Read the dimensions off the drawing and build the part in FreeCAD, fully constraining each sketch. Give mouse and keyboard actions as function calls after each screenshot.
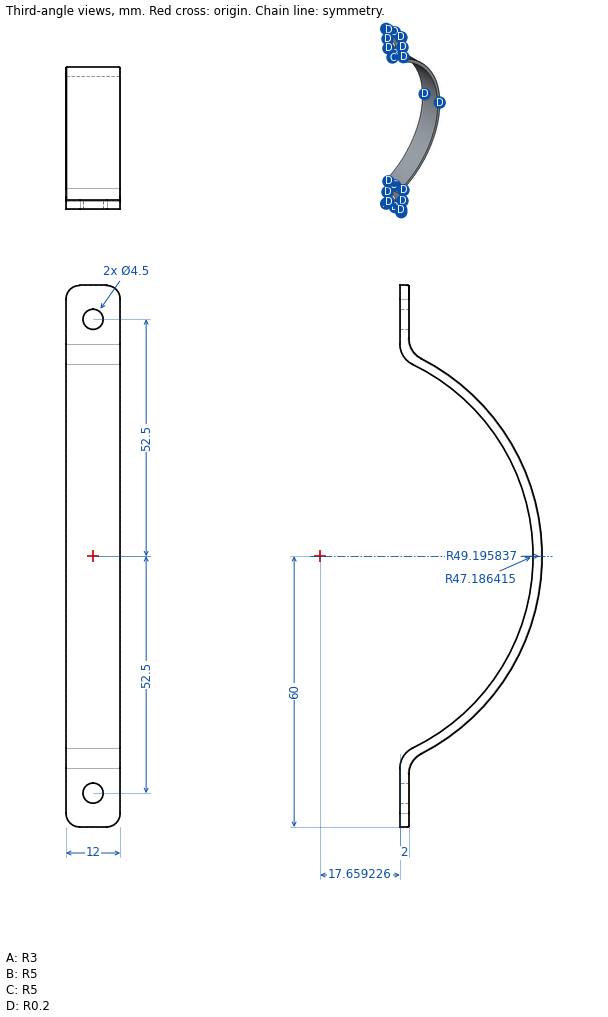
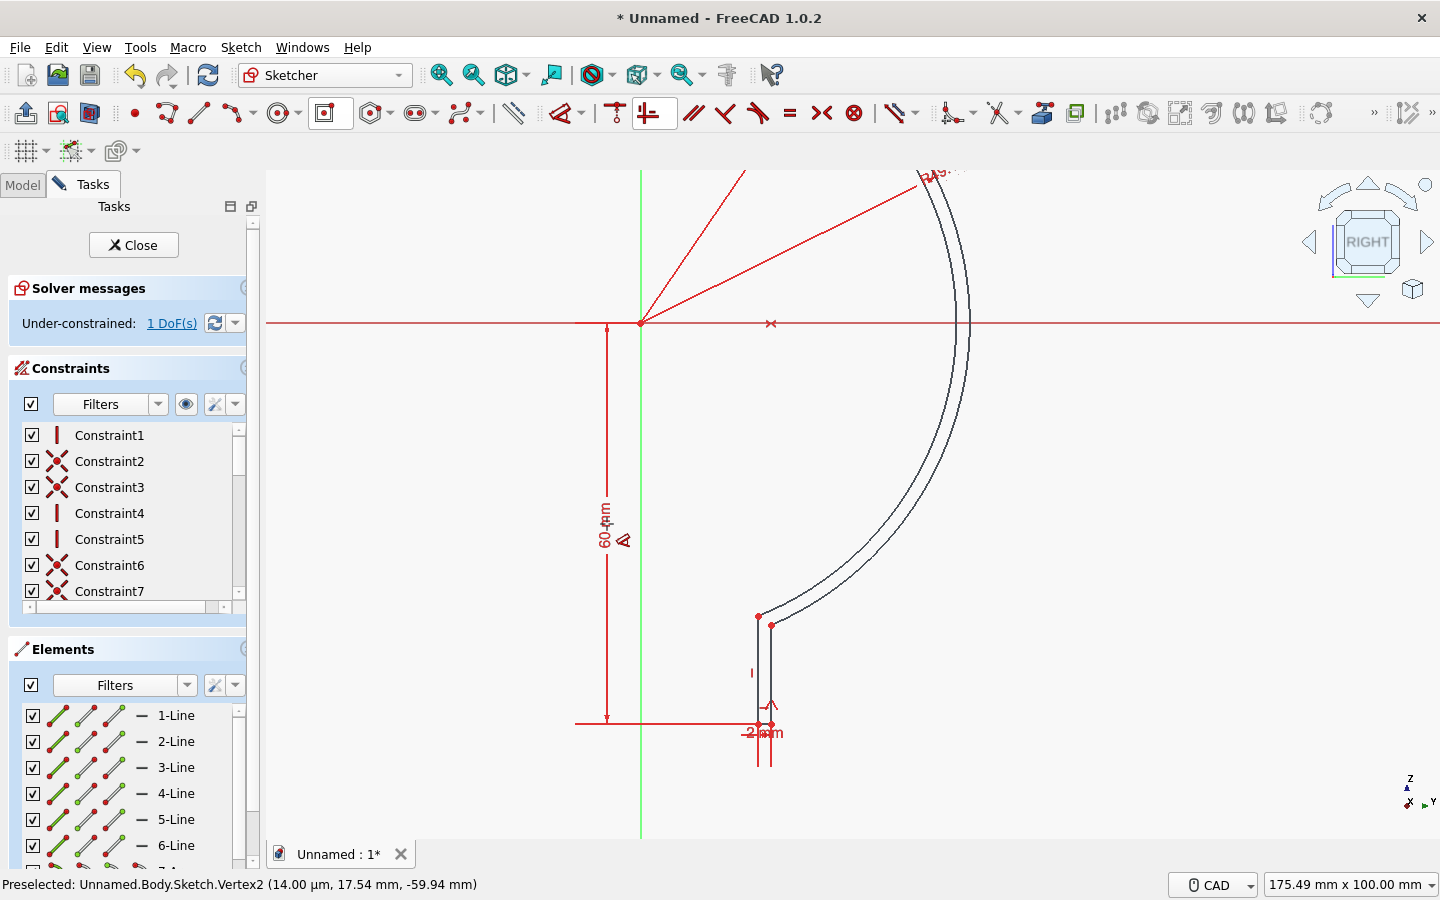
click(758, 616)
click(699, 650)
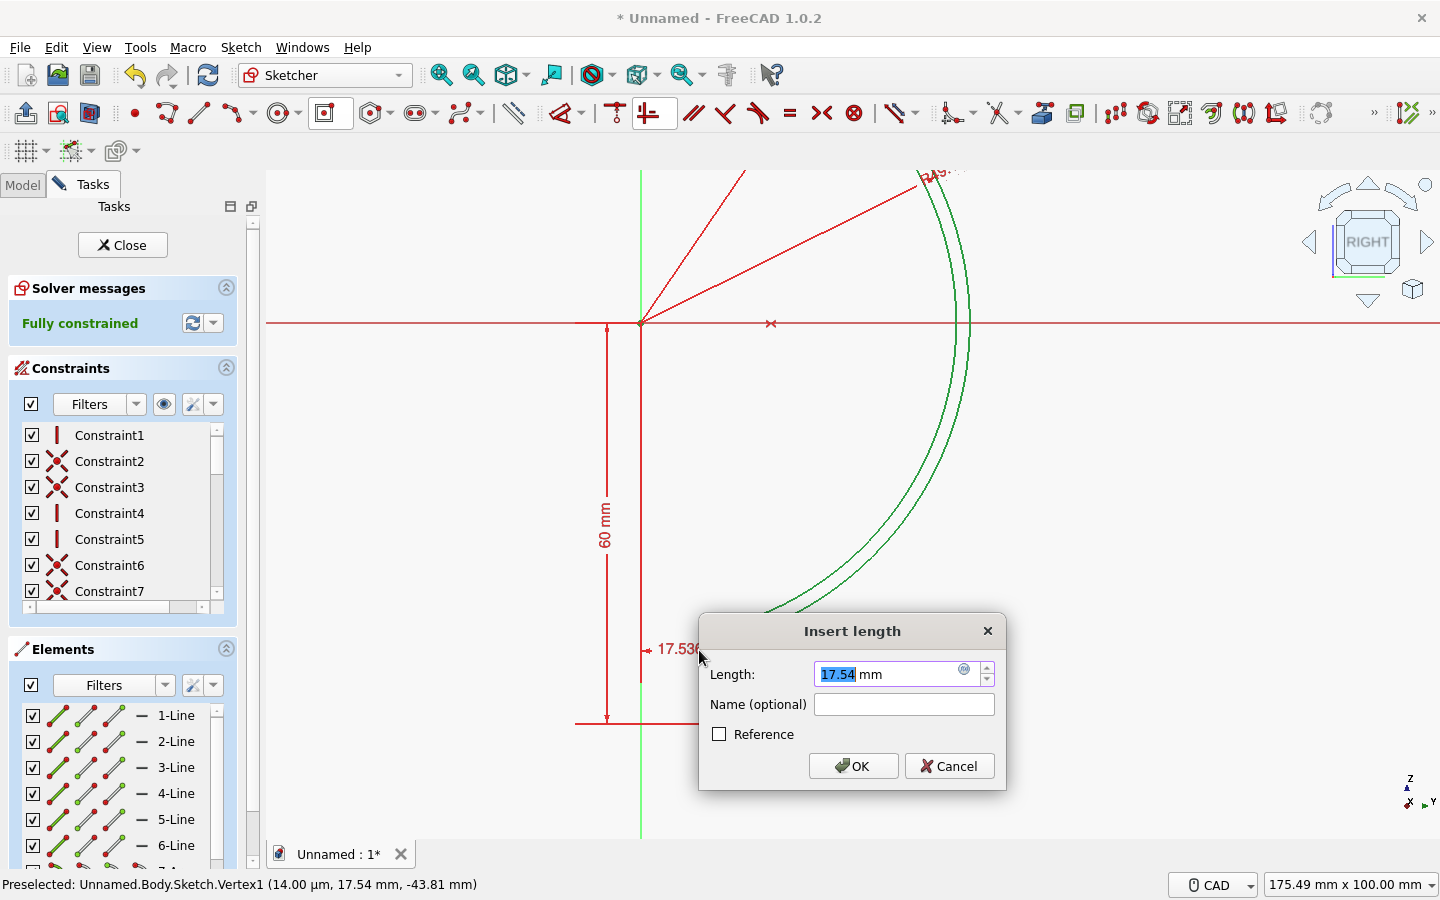
text(17.659226)
key(Return)
key(Escape)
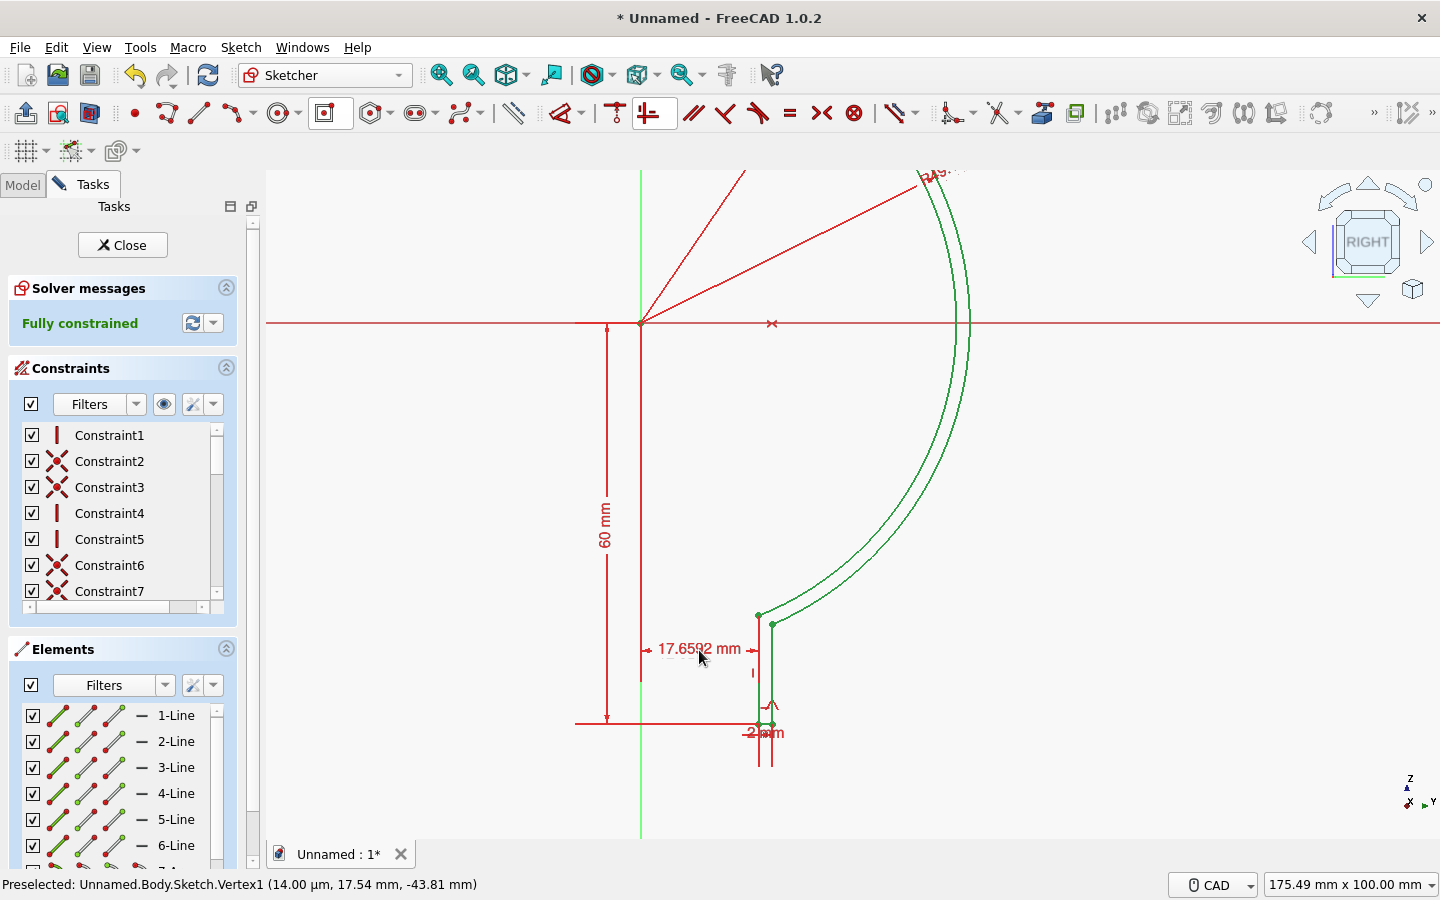
click(123, 245)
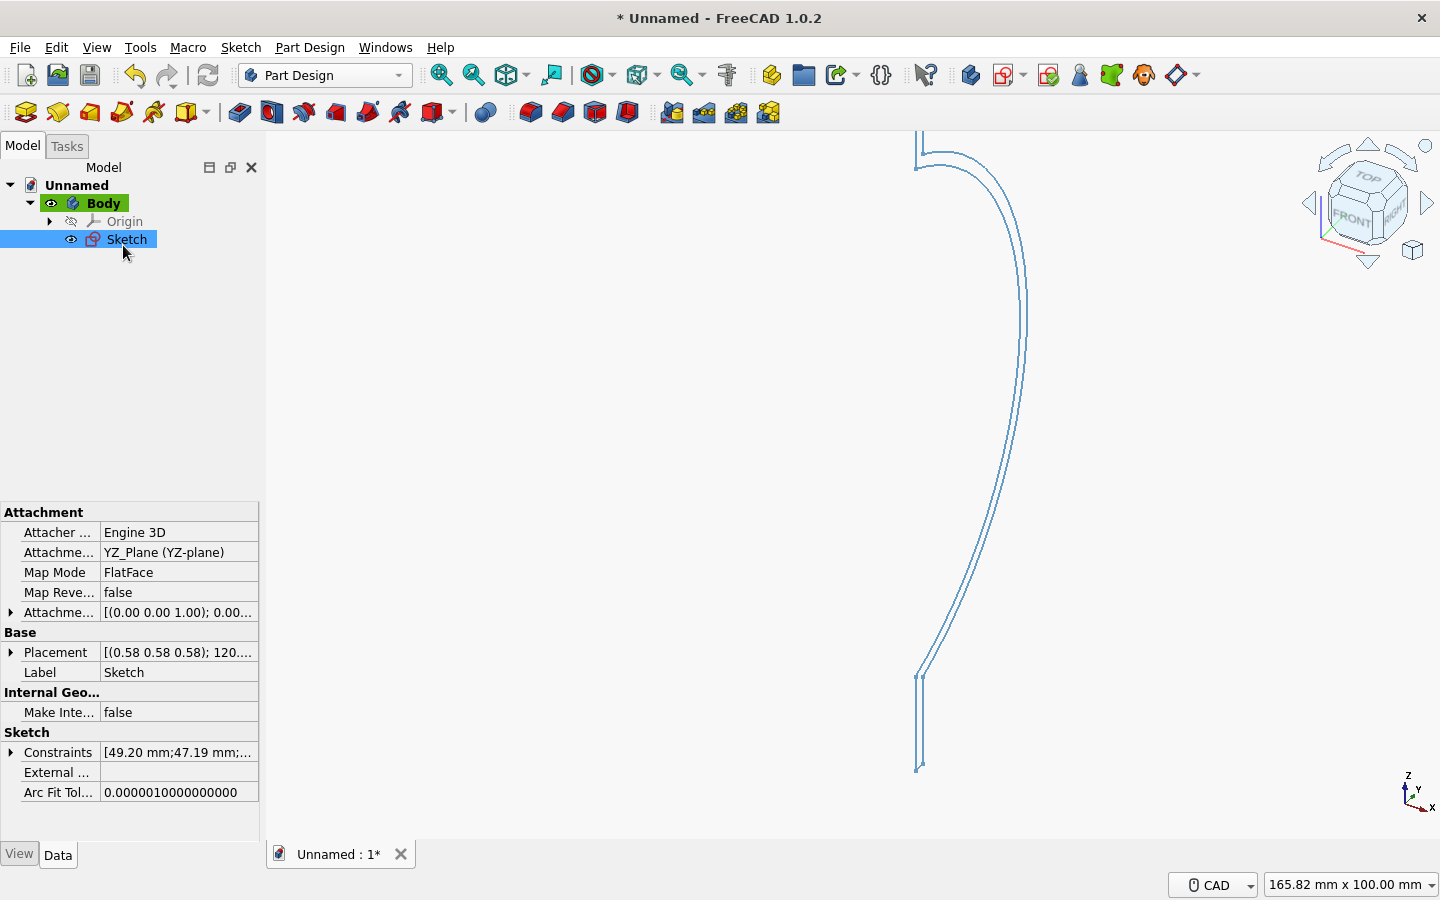
click(26, 112)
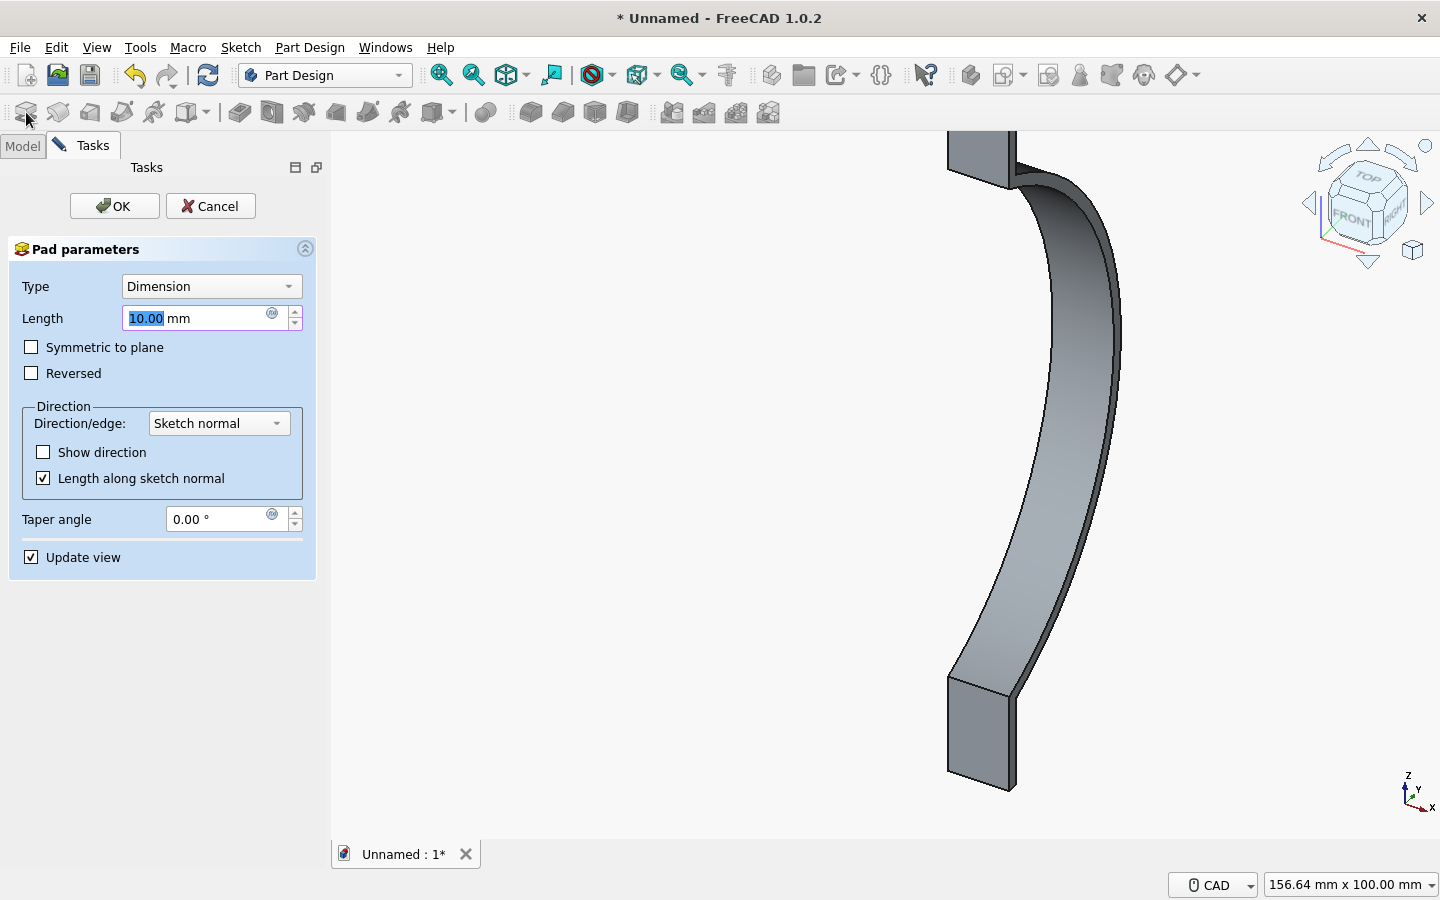
text(12)
key(Tab)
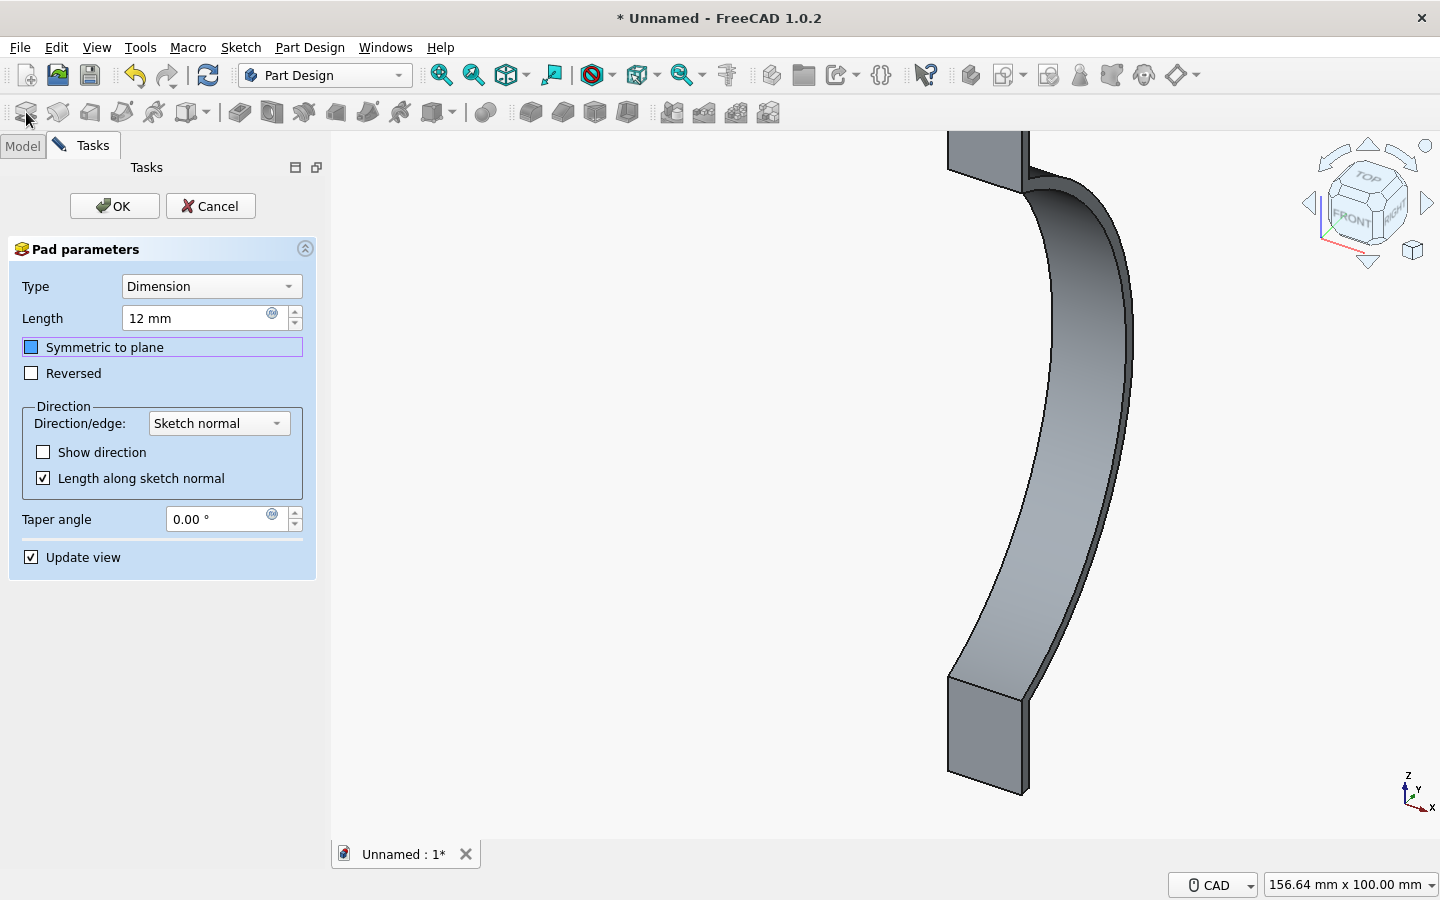
click(30, 347)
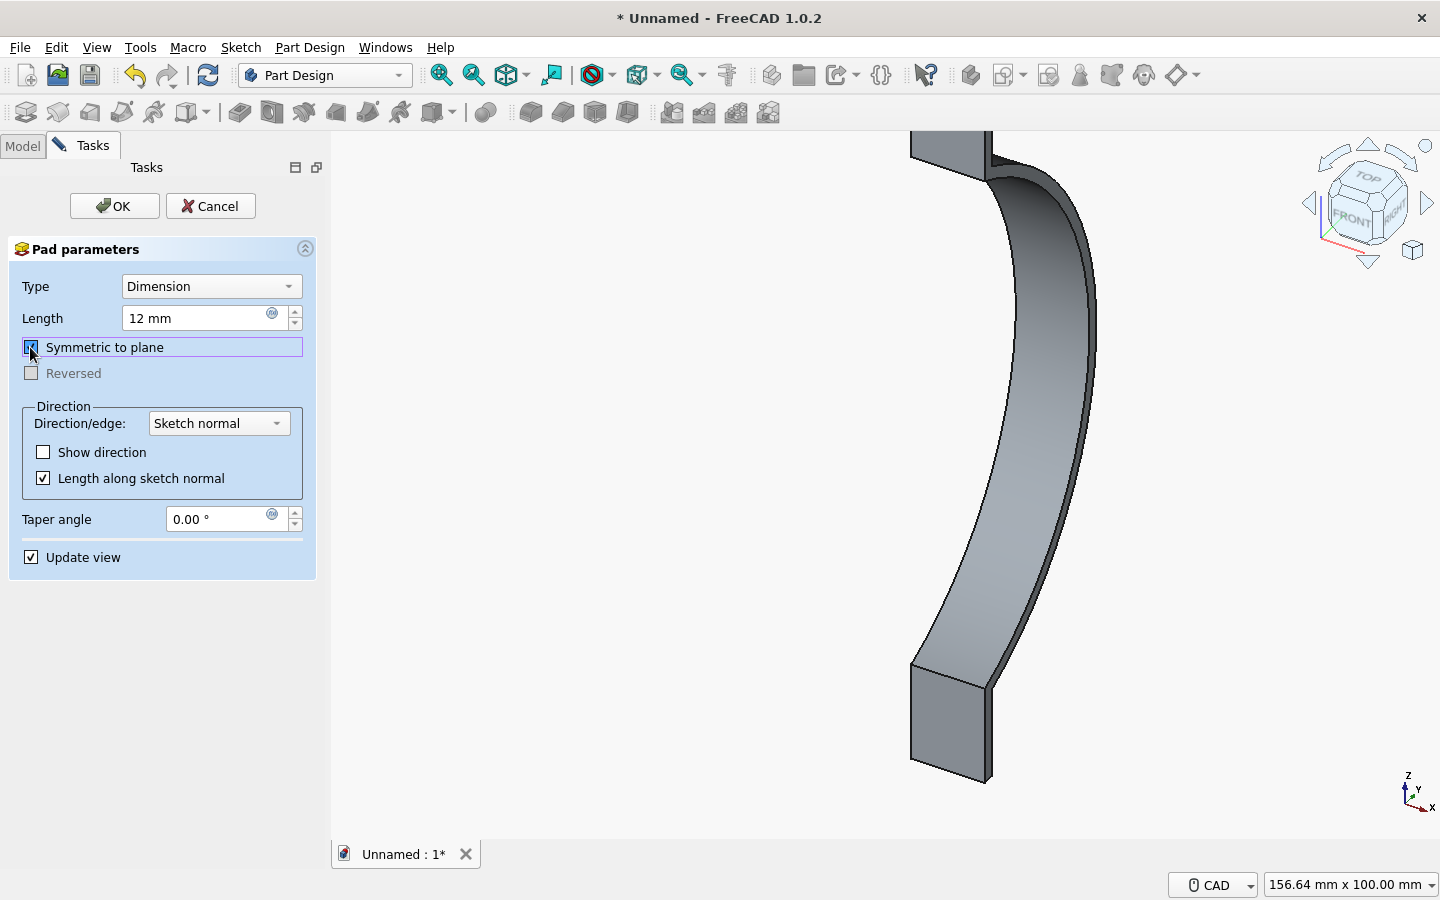
click(115, 206)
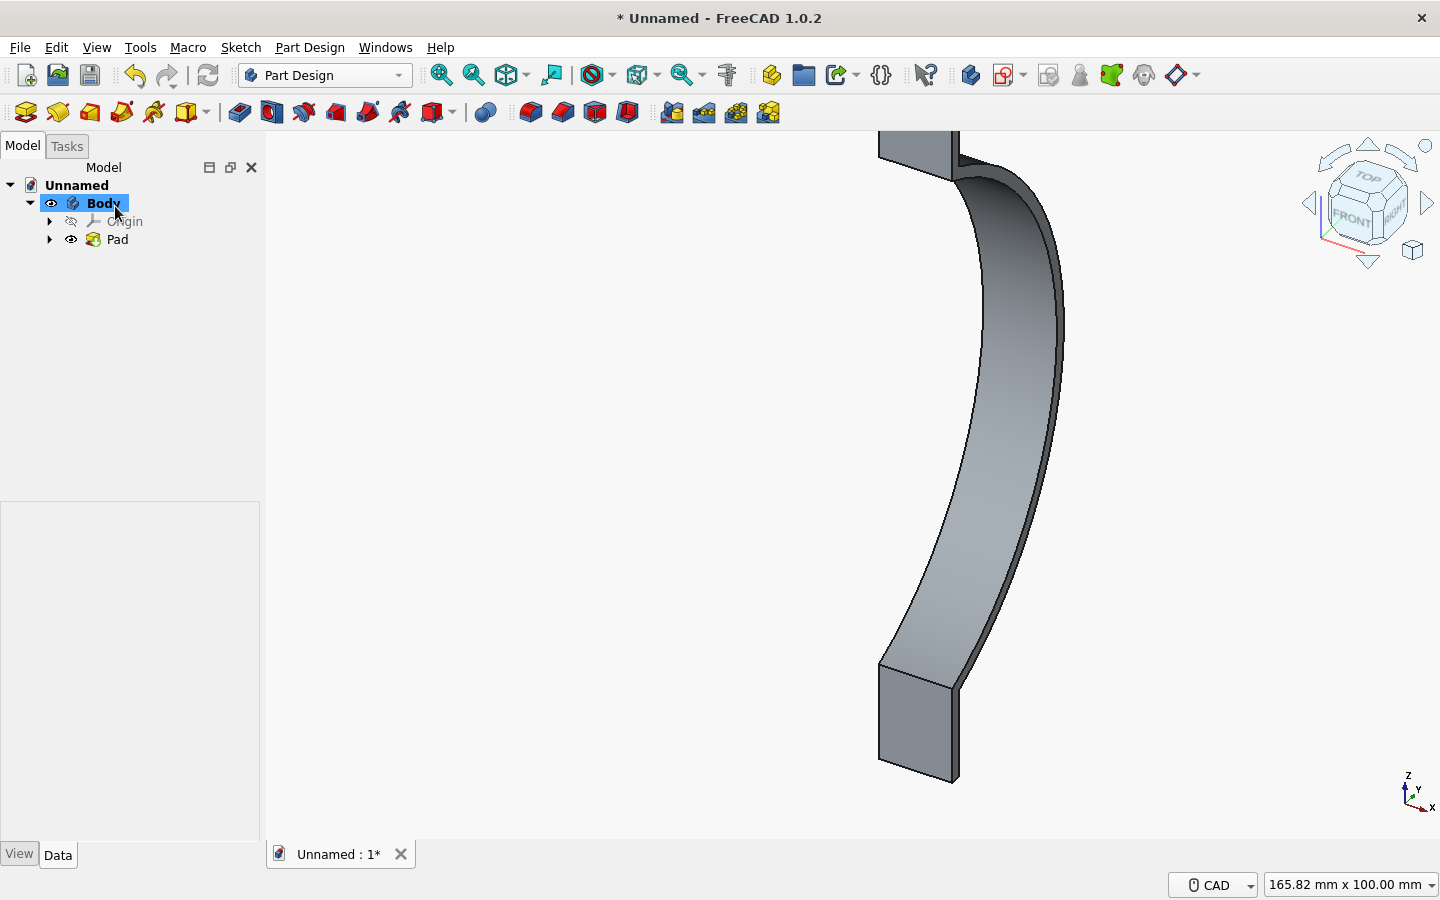
click(442, 76)